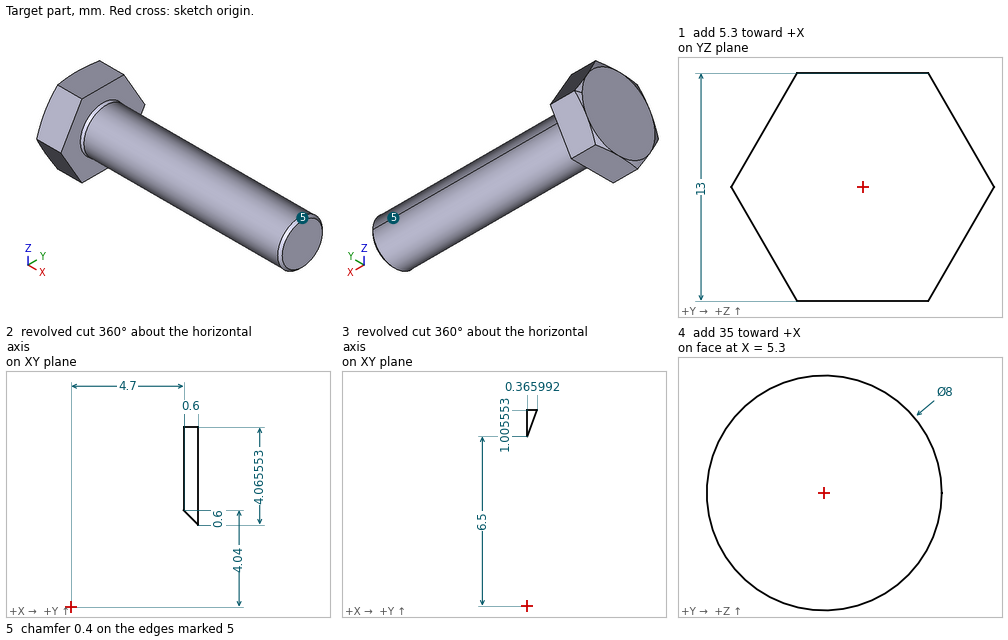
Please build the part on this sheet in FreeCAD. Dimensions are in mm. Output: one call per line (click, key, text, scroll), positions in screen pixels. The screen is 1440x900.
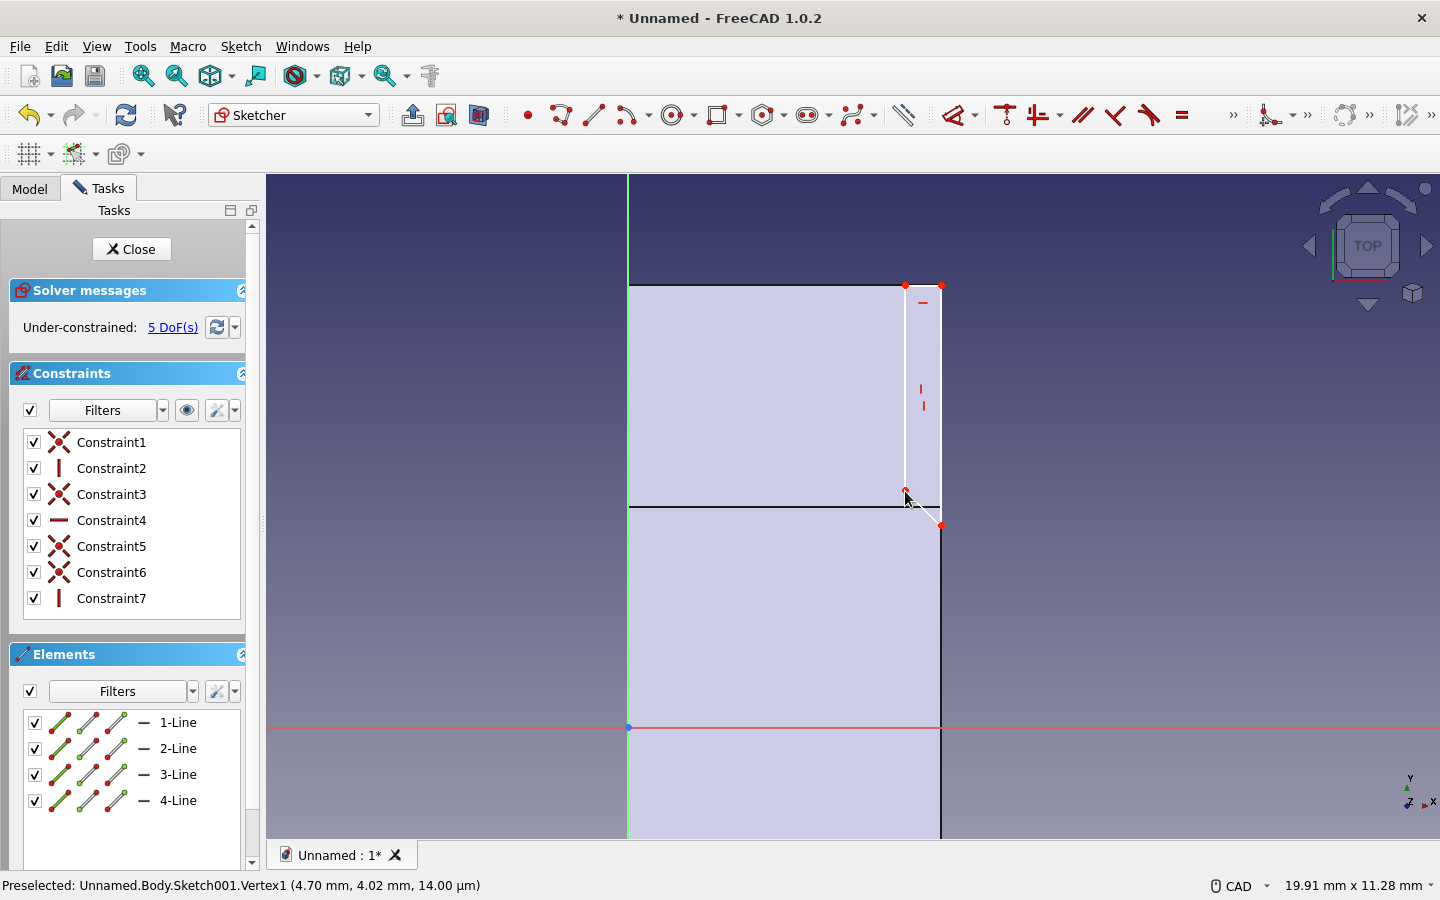
click(952, 116)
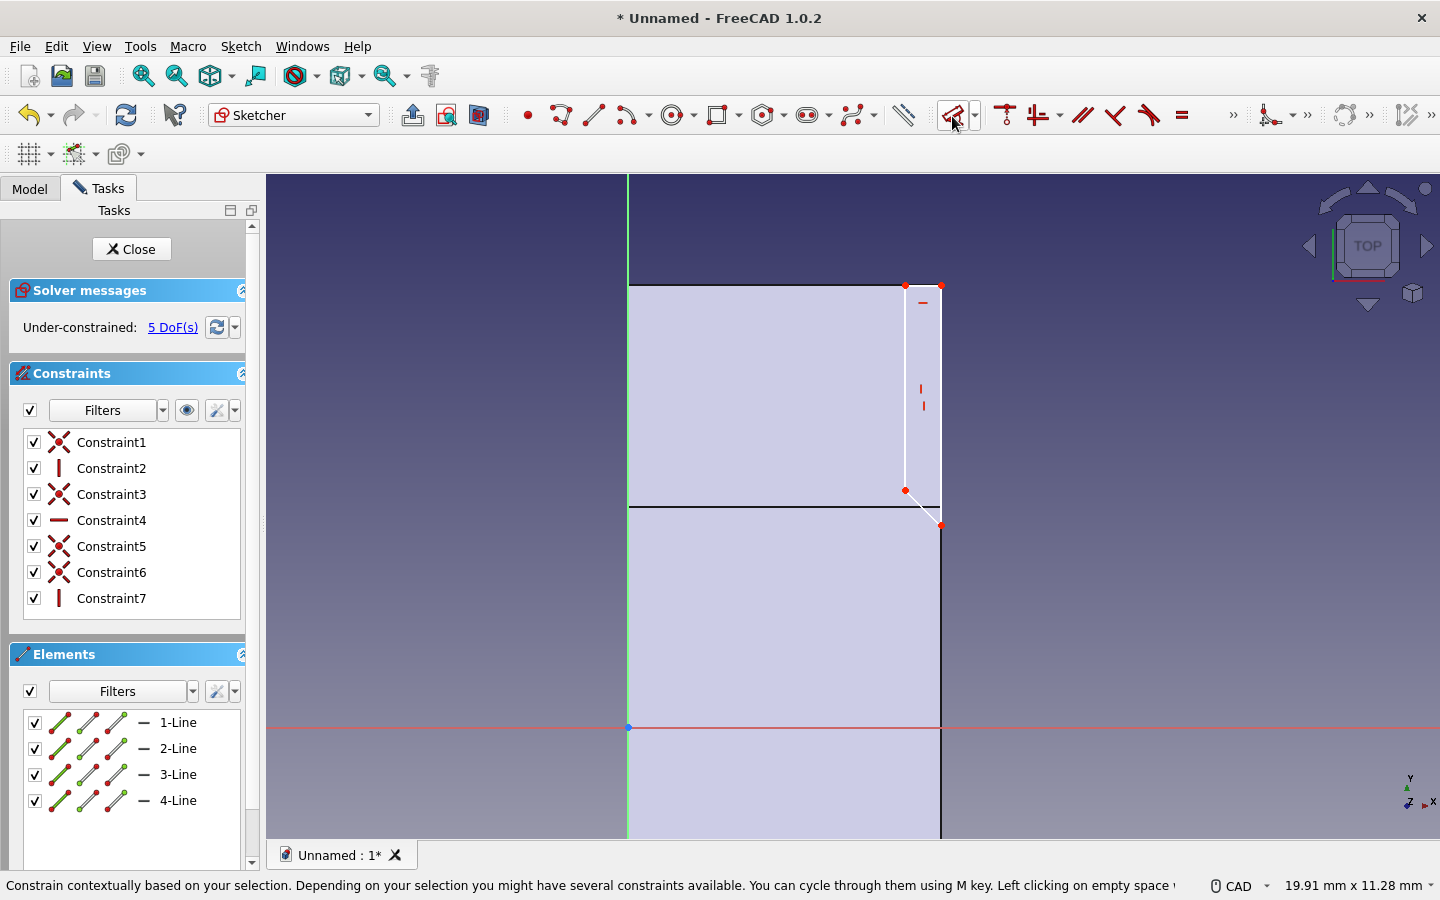
scroll(930, 286, up, 2)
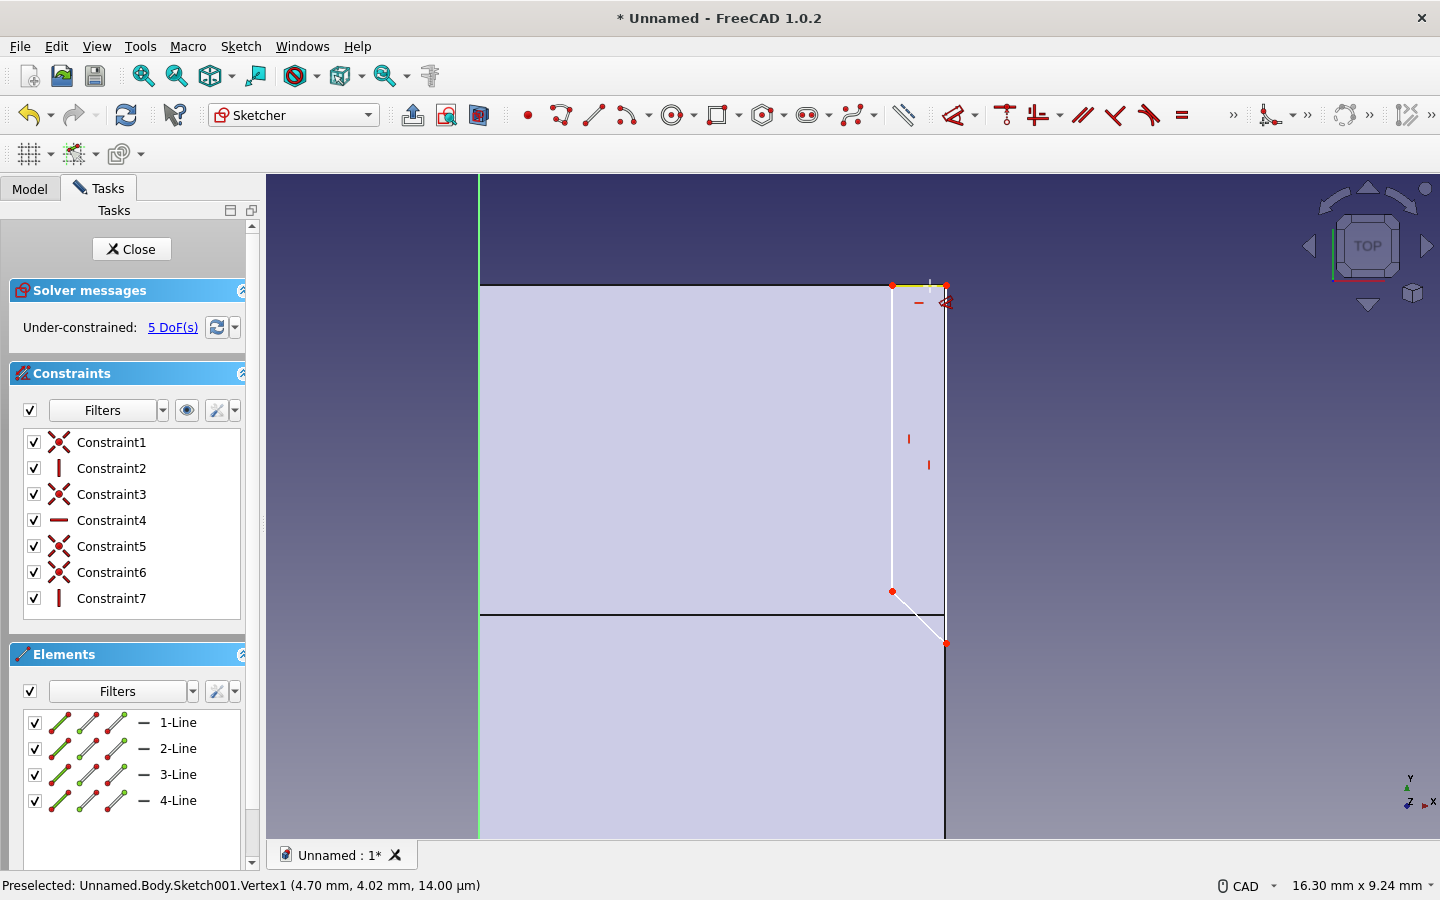
click(930, 286)
click(919, 252)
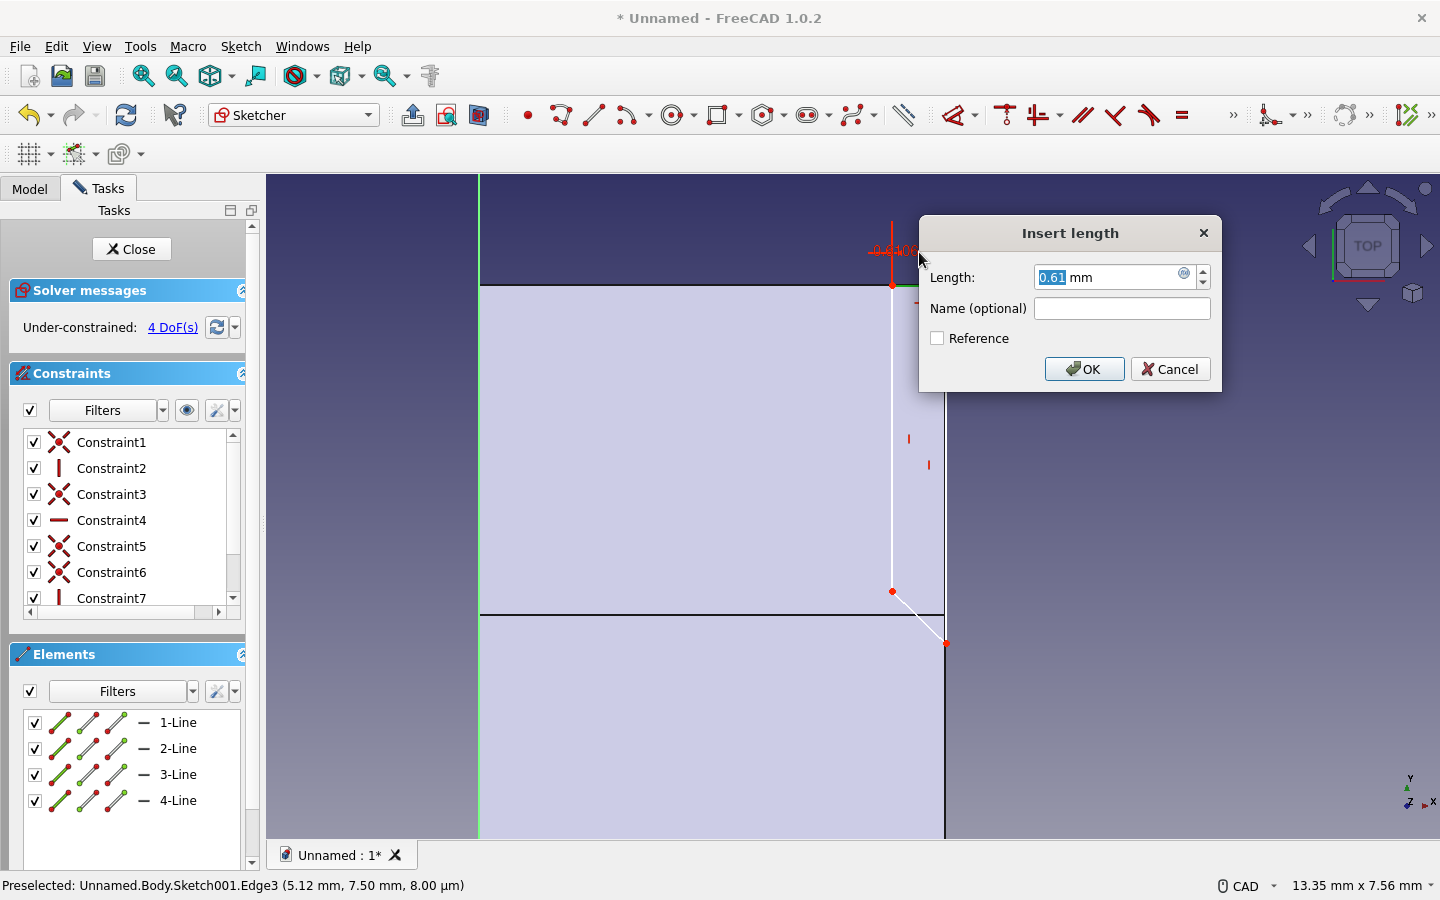
text(0.6)
key(Return)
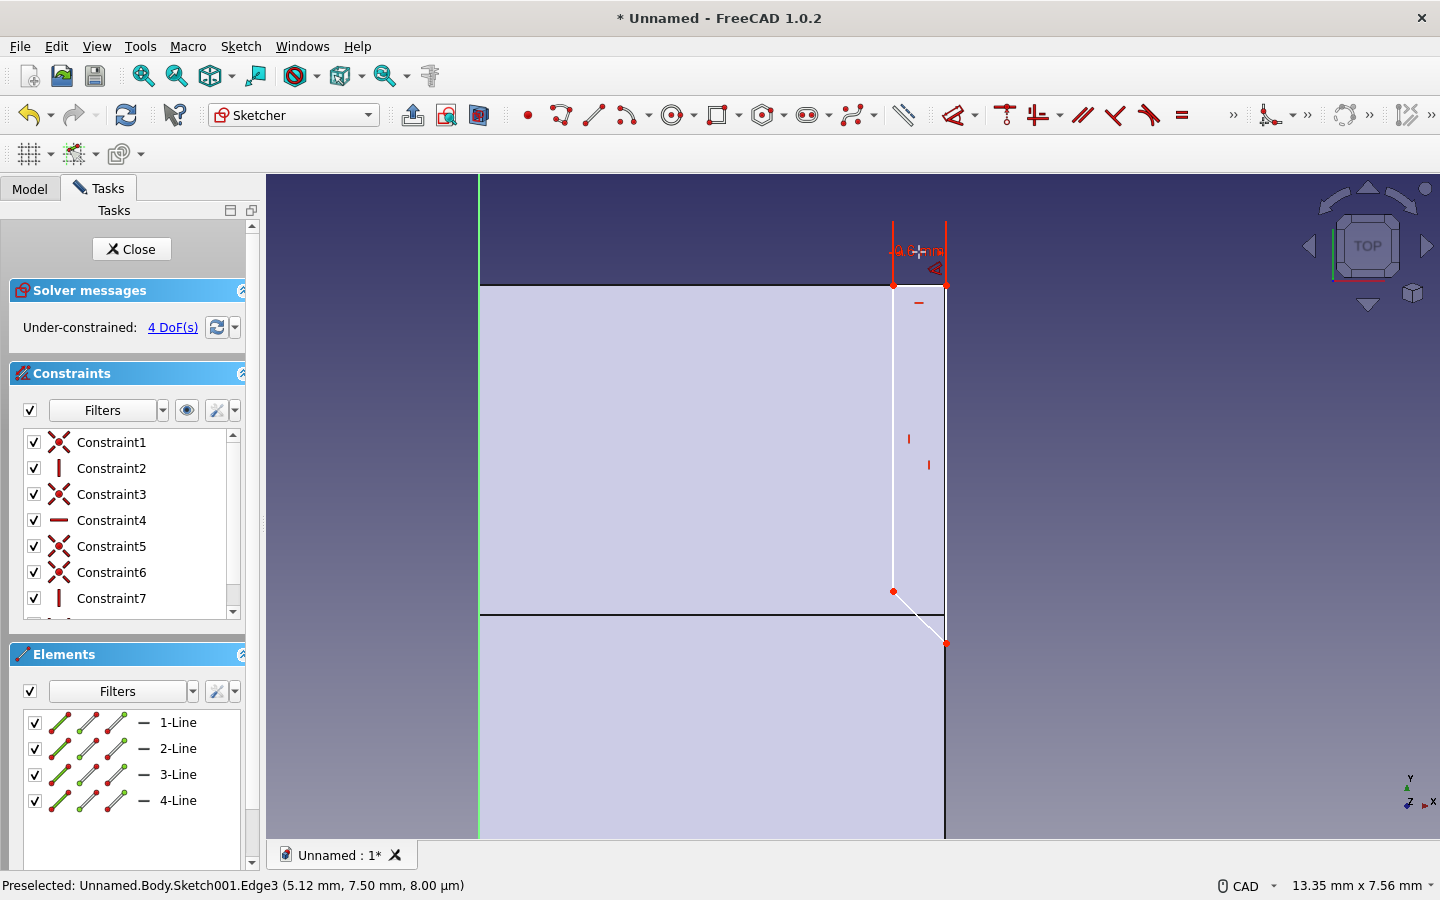
click(893, 592)
click(686, 558)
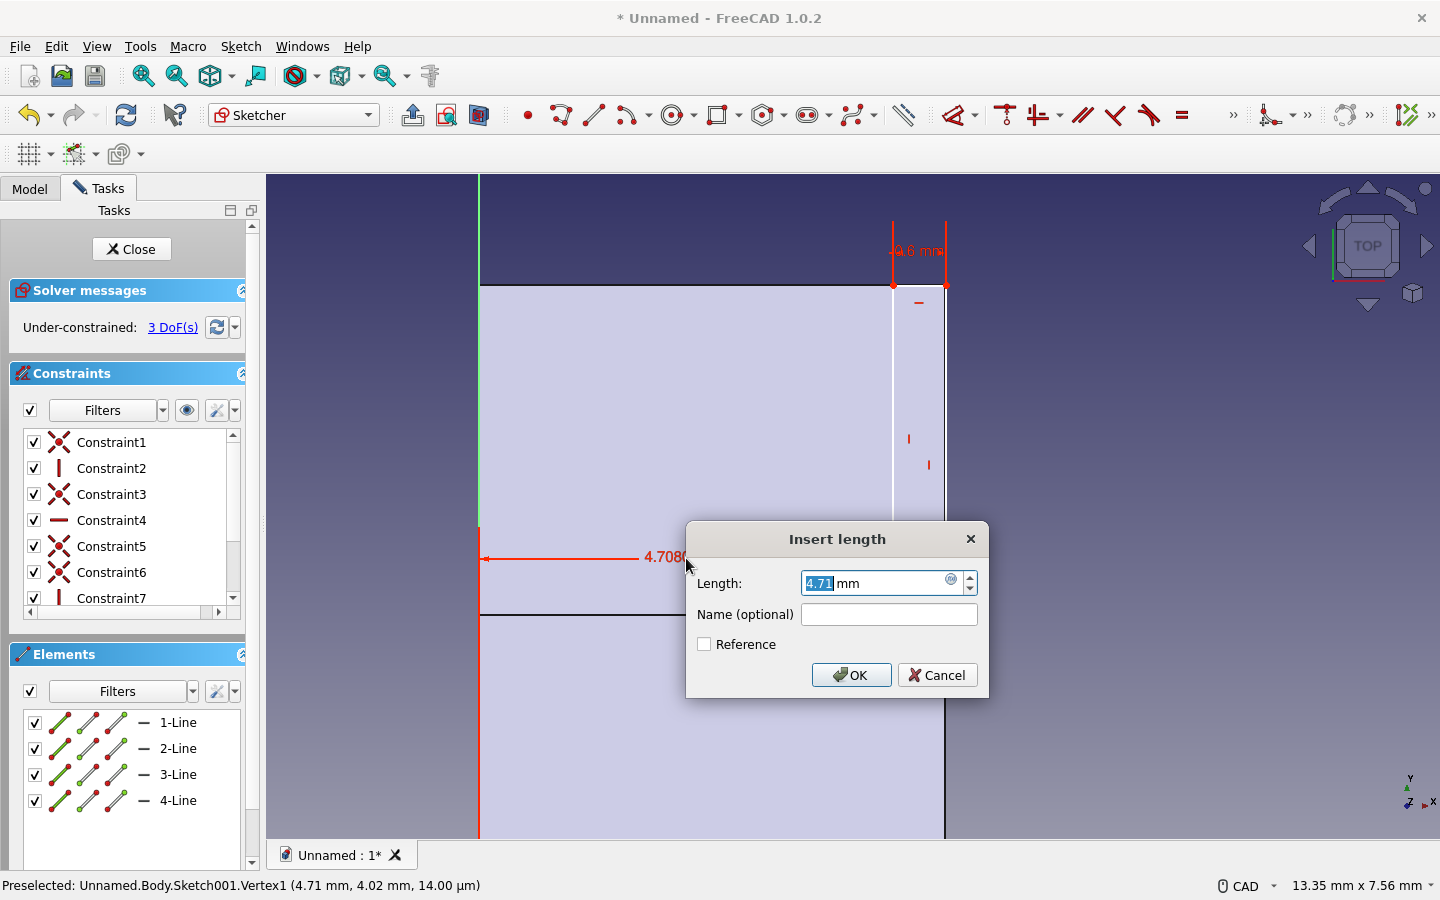
text(4.7)
key(Return)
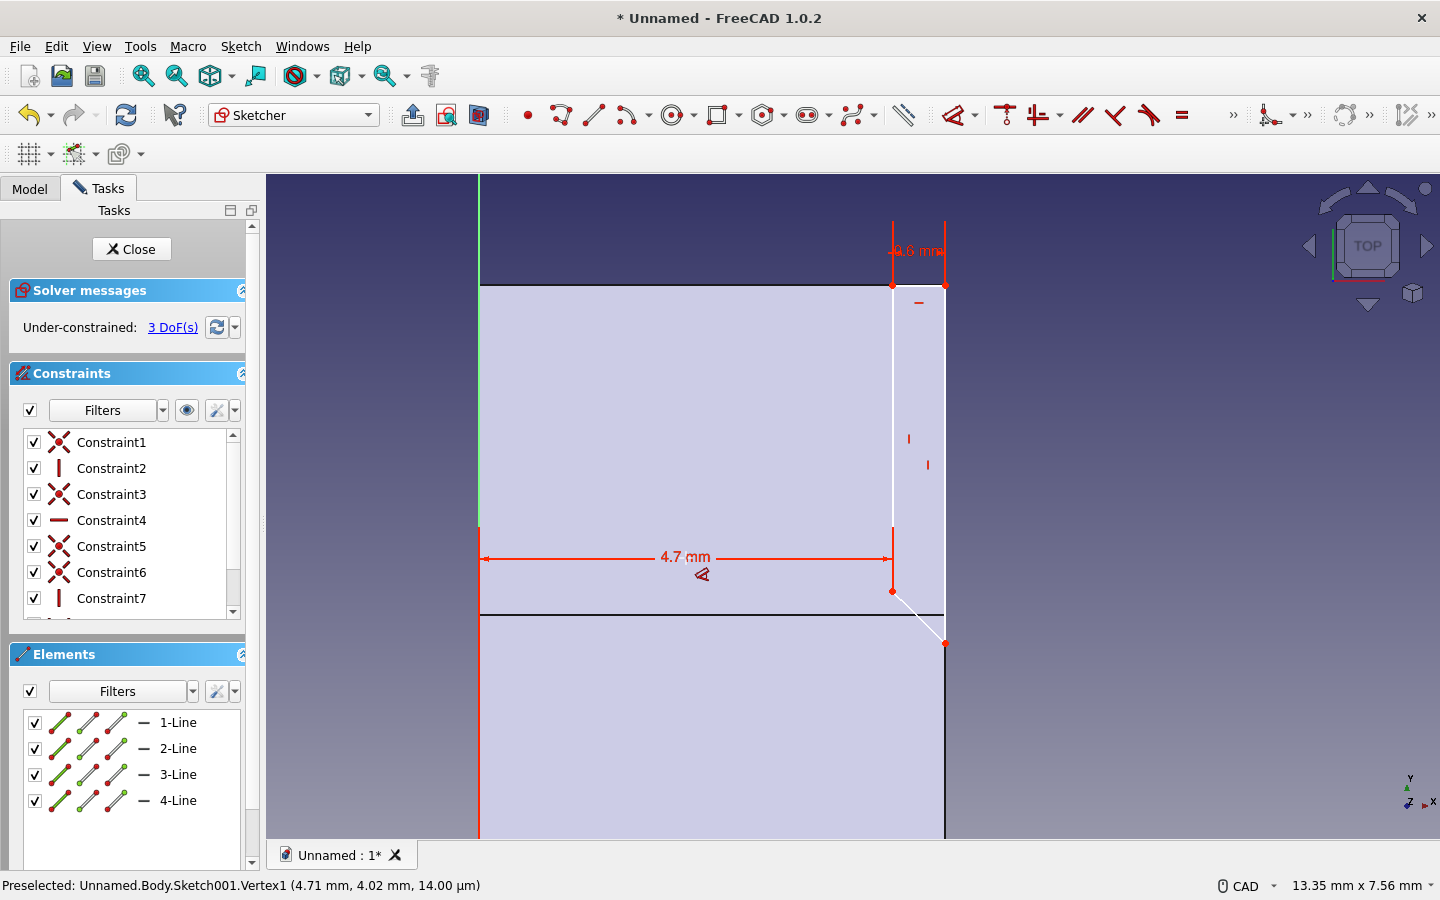
click(908, 607)
click(979, 618)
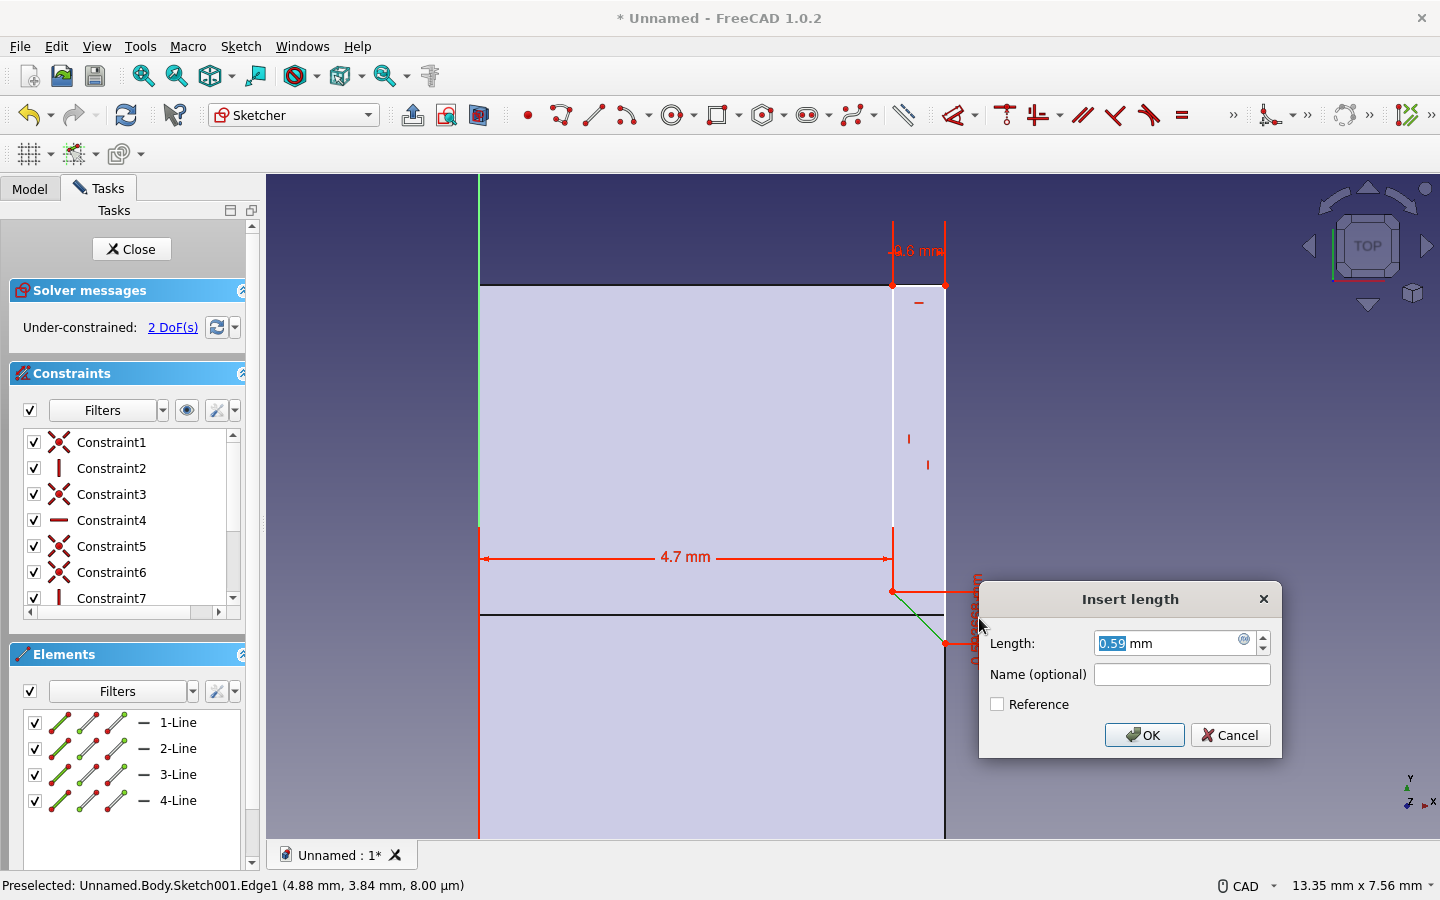
text(0.6)
key(Return)